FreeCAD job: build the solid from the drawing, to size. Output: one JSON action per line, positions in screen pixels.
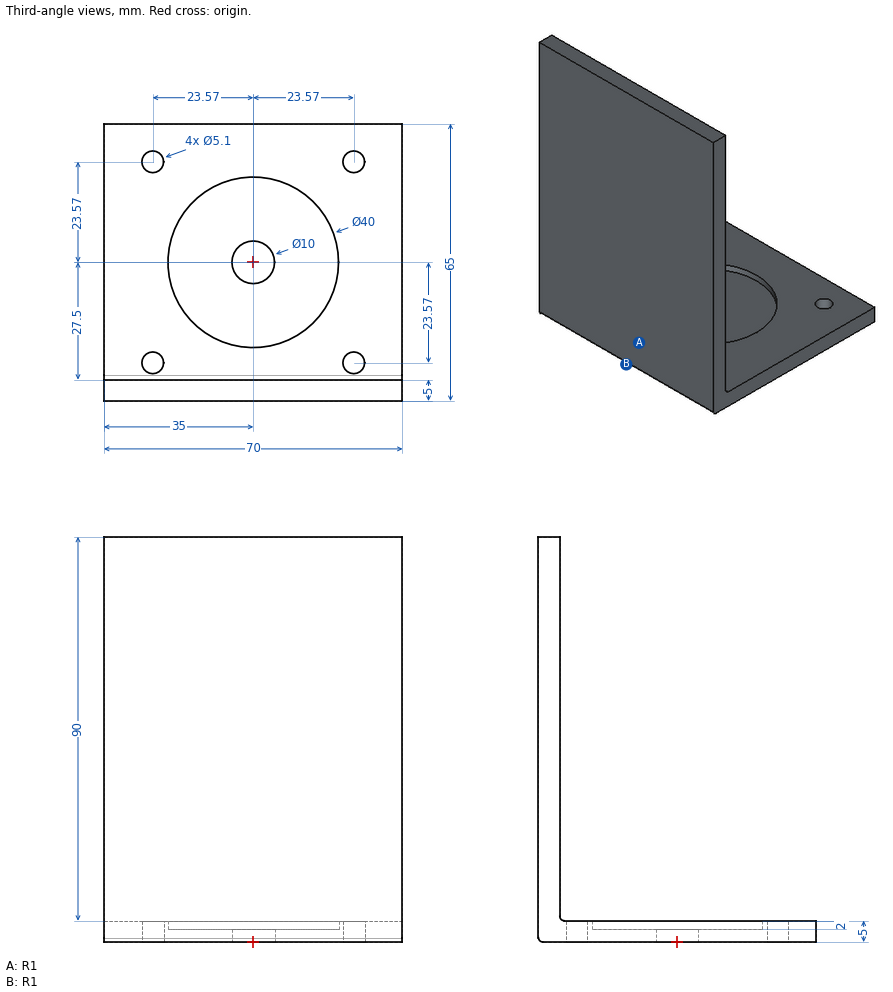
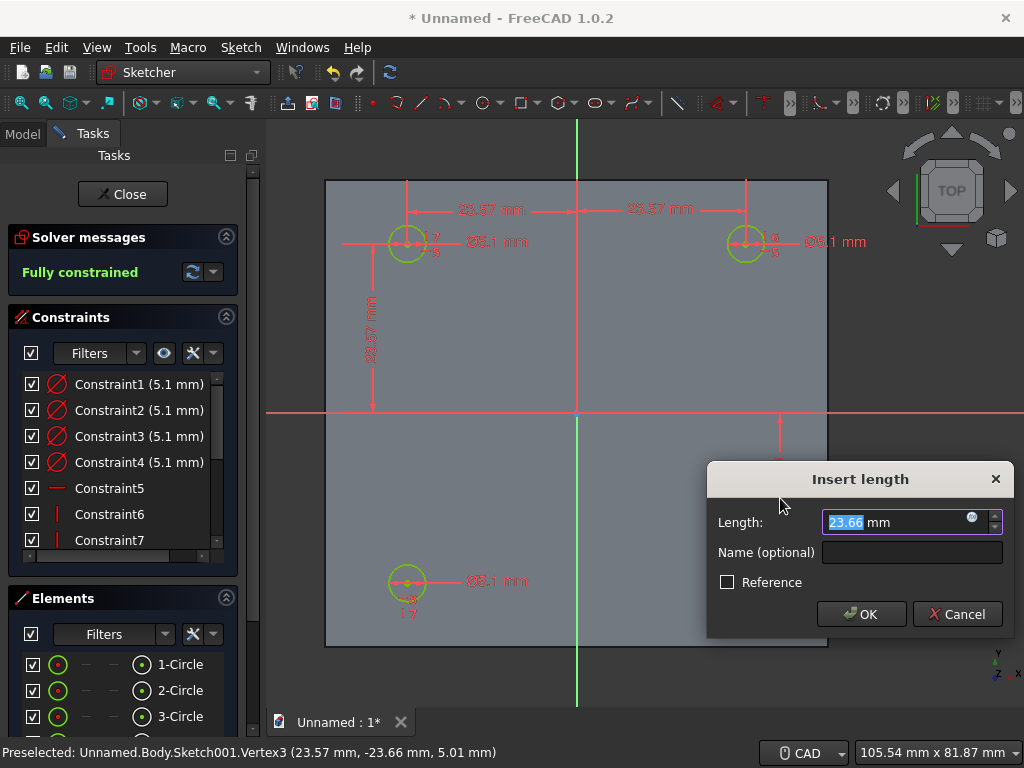
{"action": "type", "text": "23.57"}
{"action": "key", "text": "Return"}
{"action": "key", "text": "Escape"}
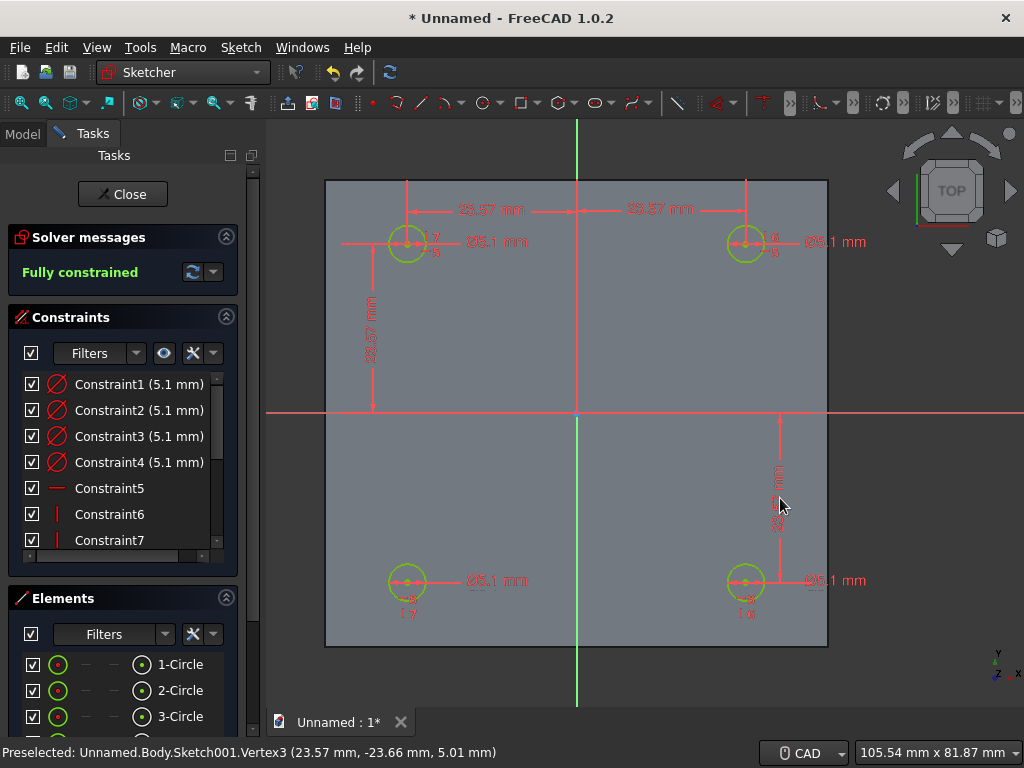
{"action": "left_click", "coordinate": [123, 194]}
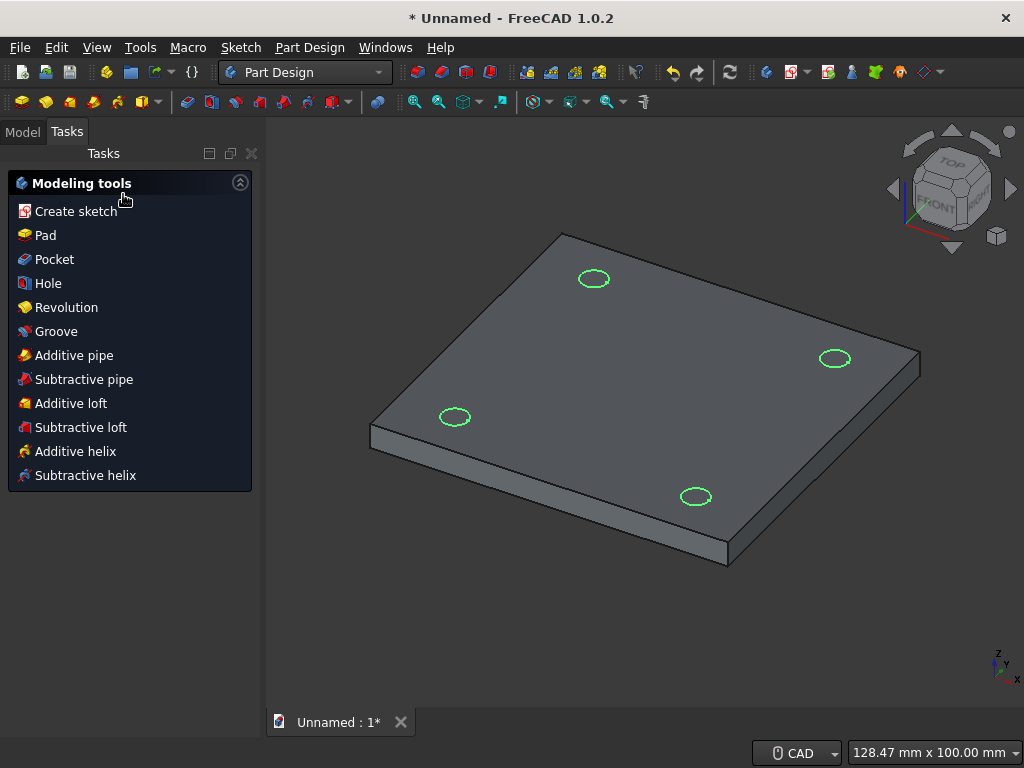
{"action": "left_click", "coordinate": [188, 102]}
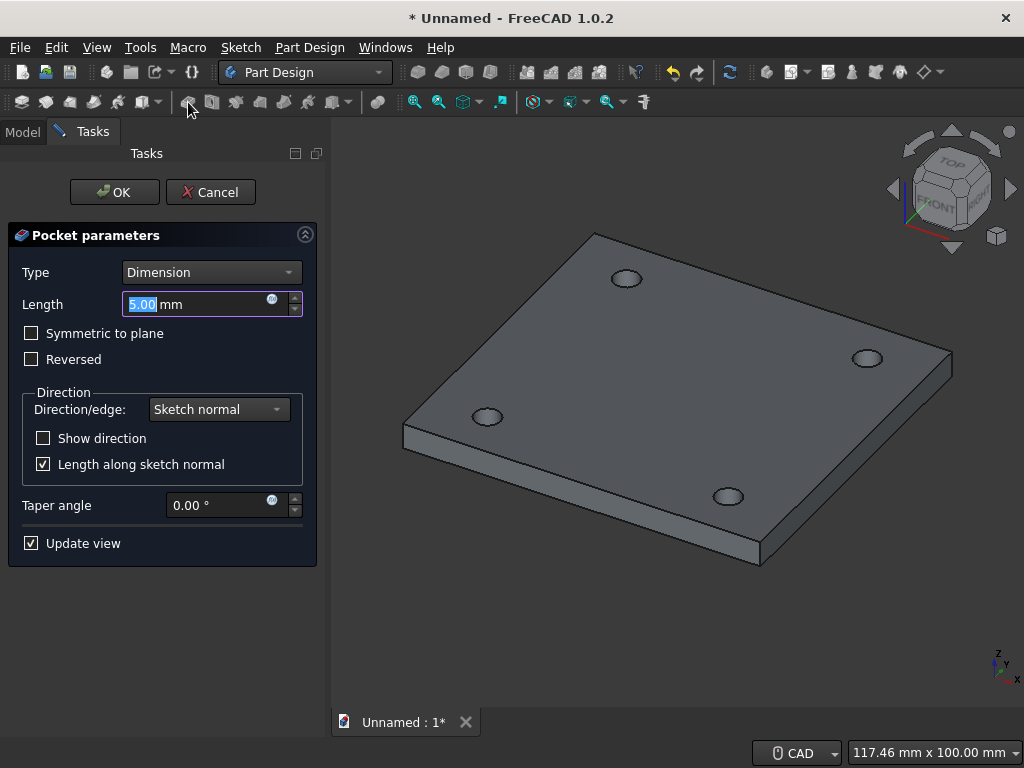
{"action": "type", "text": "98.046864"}
{"action": "key", "text": "Tab"}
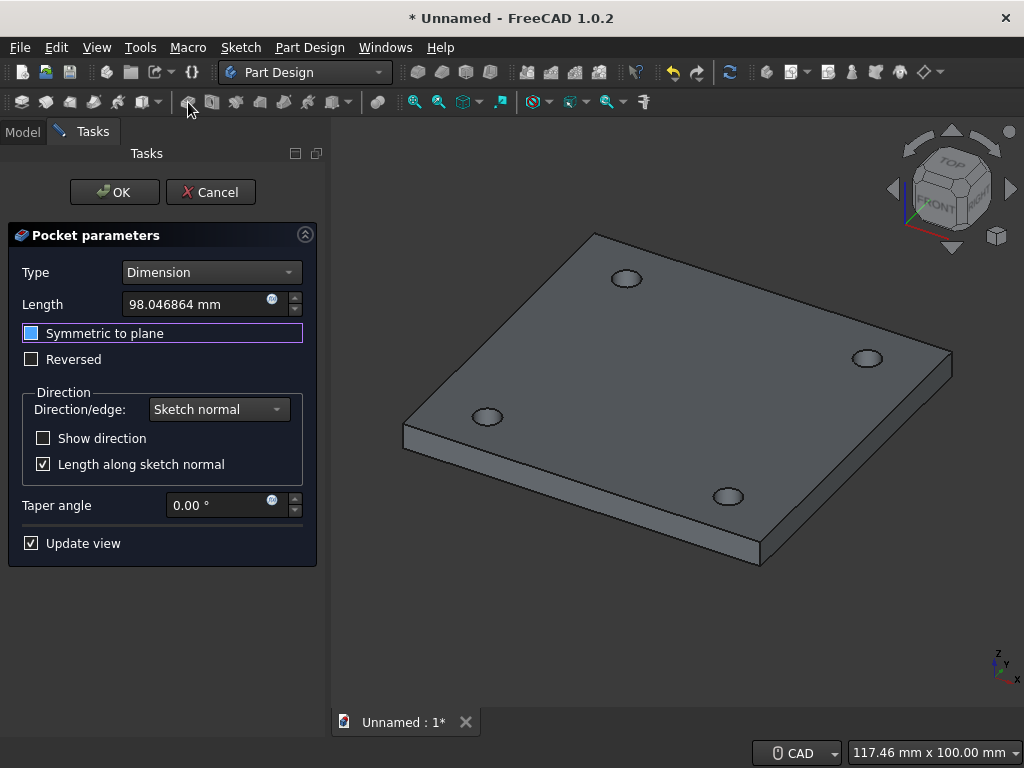
{"action": "left_click", "coordinate": [30, 333]}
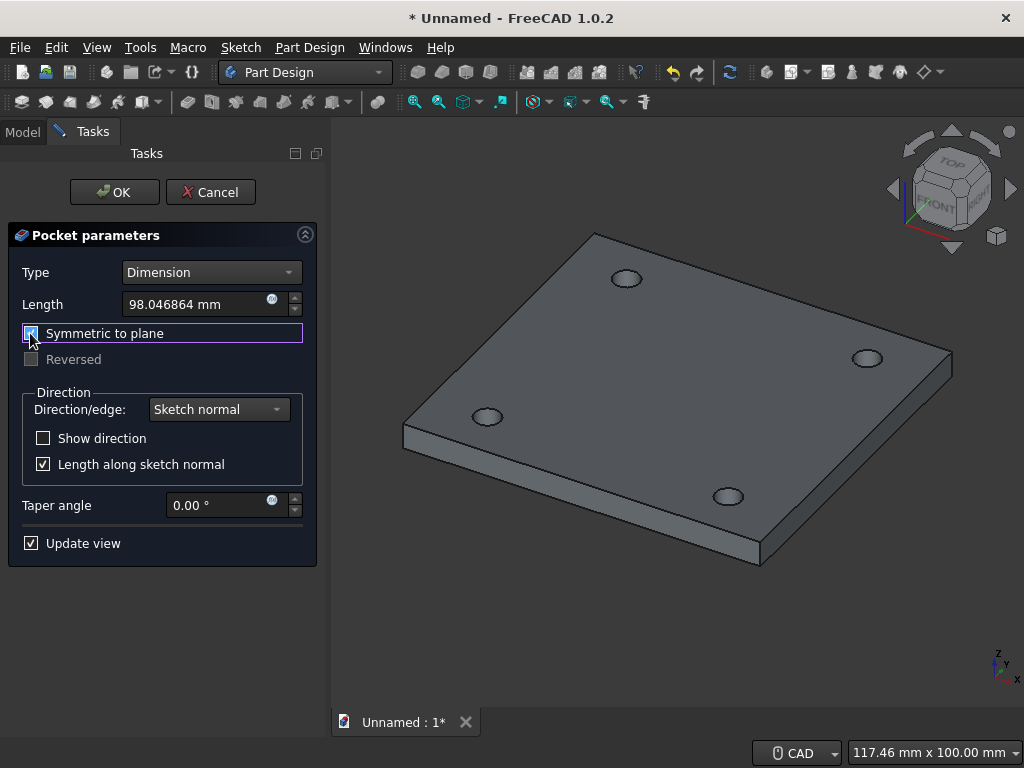
{"action": "left_click", "coordinate": [115, 192]}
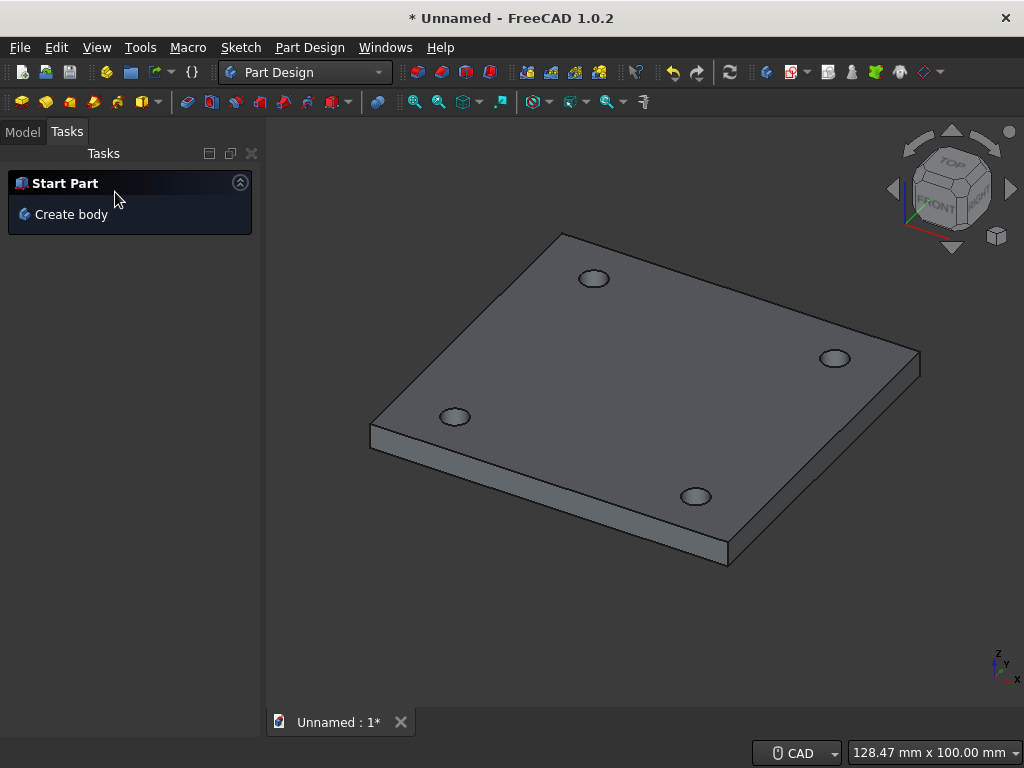
{"action": "left_click", "coordinate": [645, 387]}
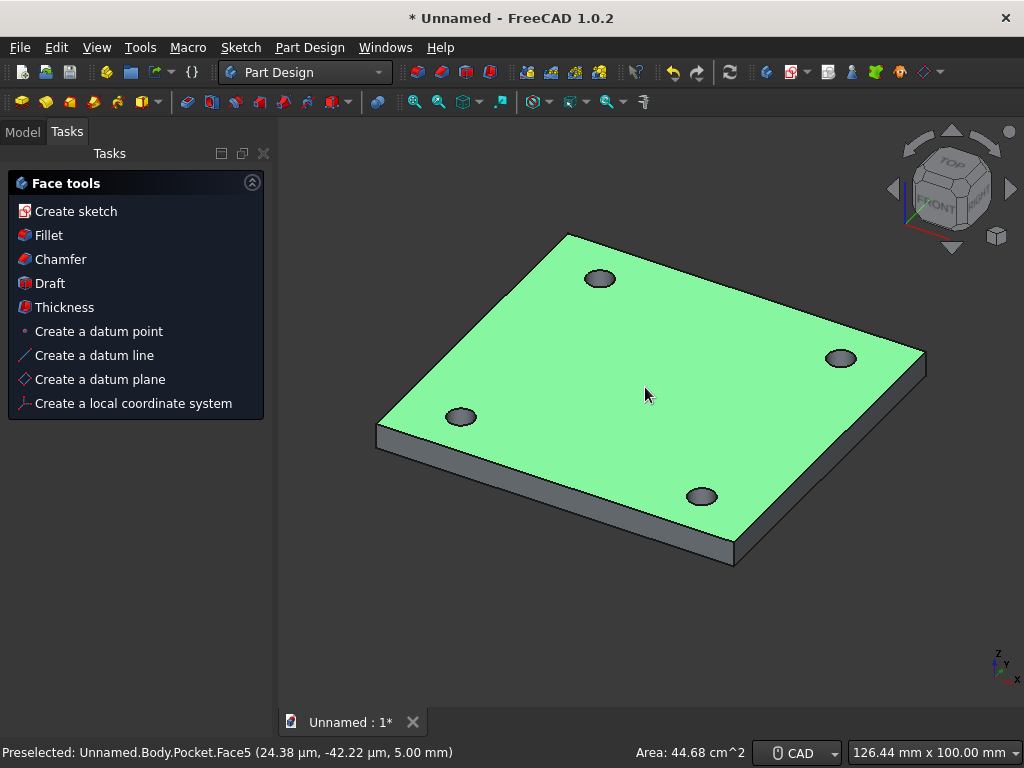
{"action": "left_click", "coordinate": [792, 72]}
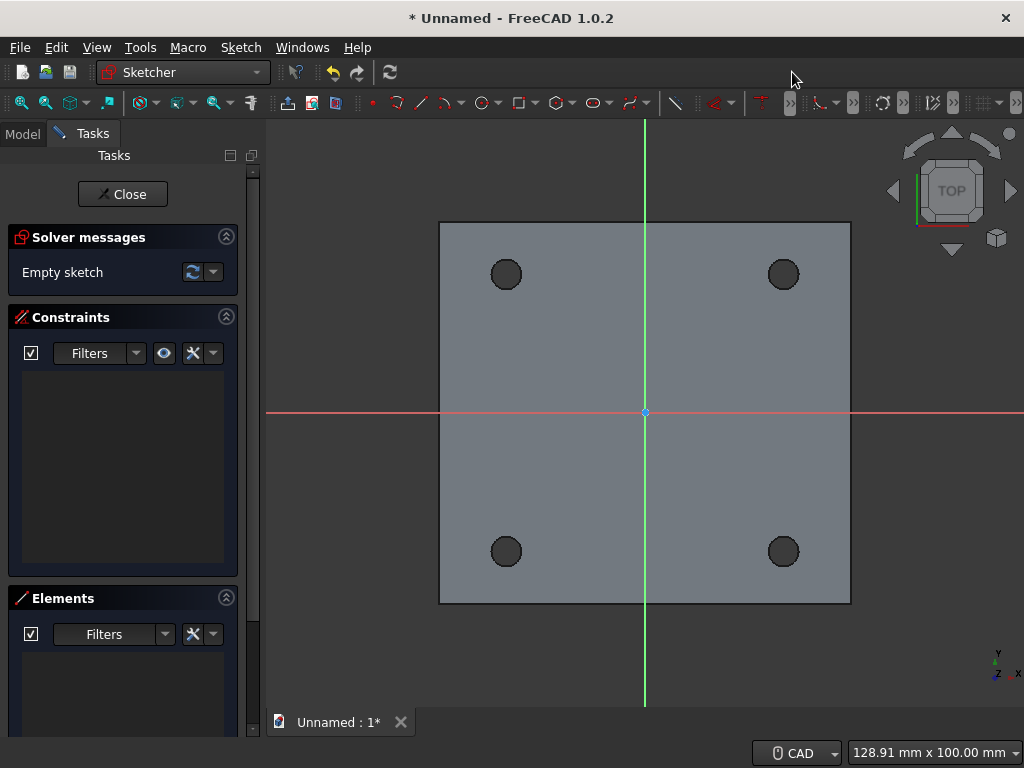
{"action": "scroll", "coordinate": [294, 147], "scroll_direction": "down", "scroll_amount": 1}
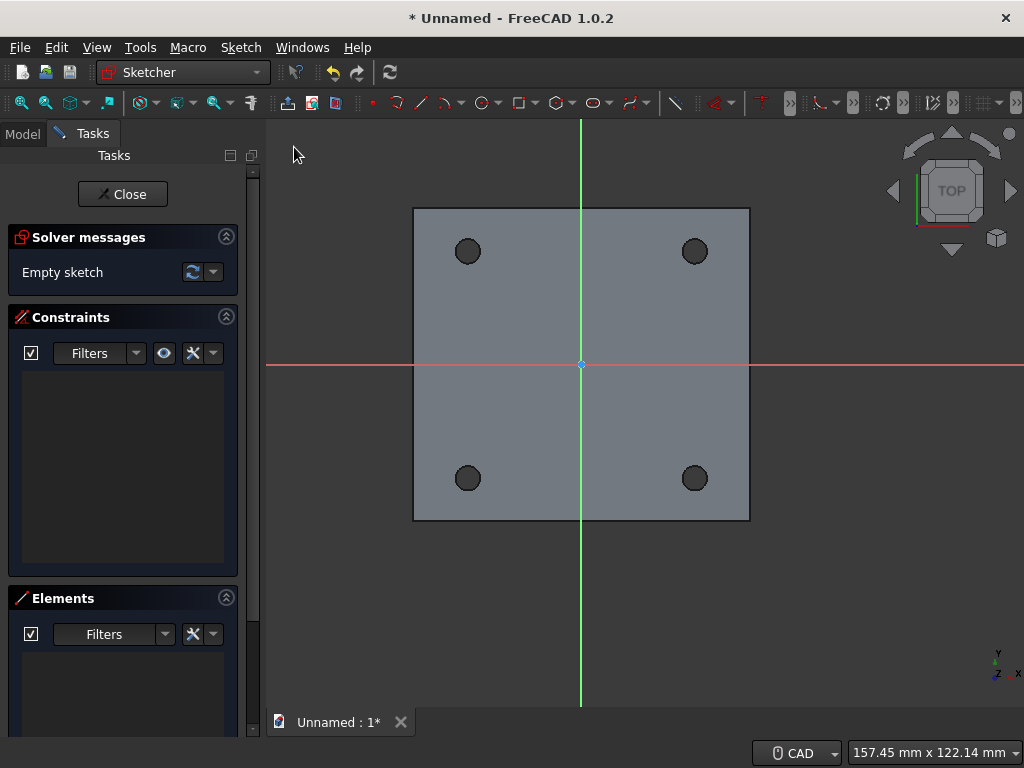
{"action": "left_click", "coordinate": [520, 104]}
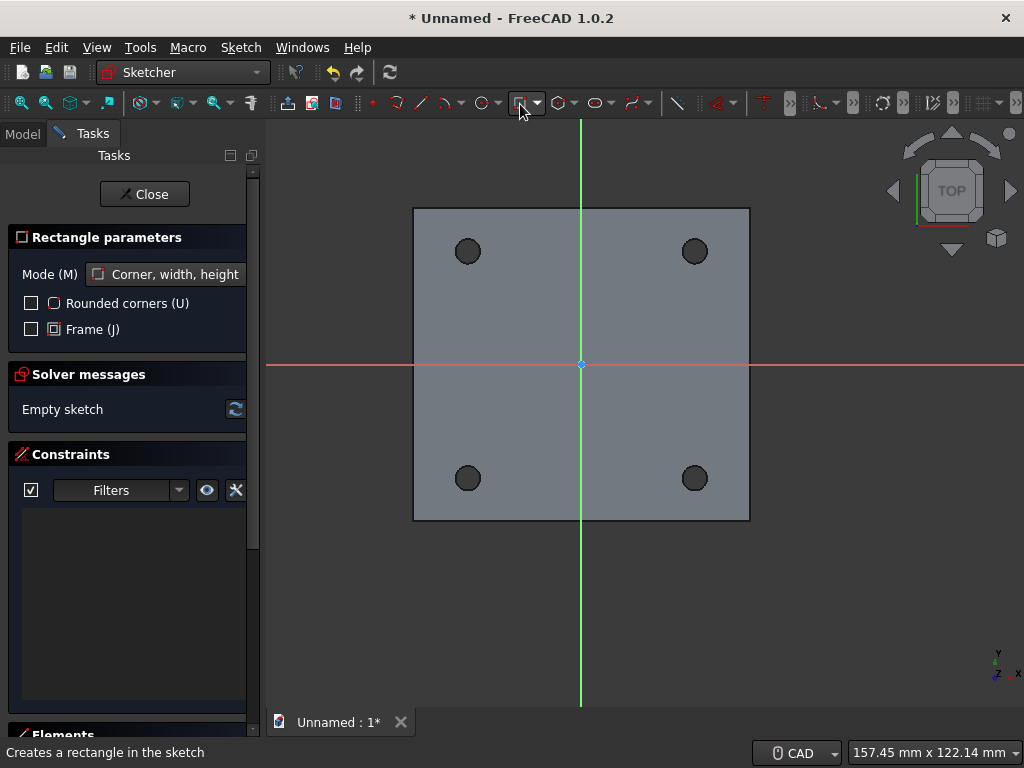
{"action": "left_click", "coordinate": [413, 497]}
{"action": "mouse_move", "coordinate": [750, 521]}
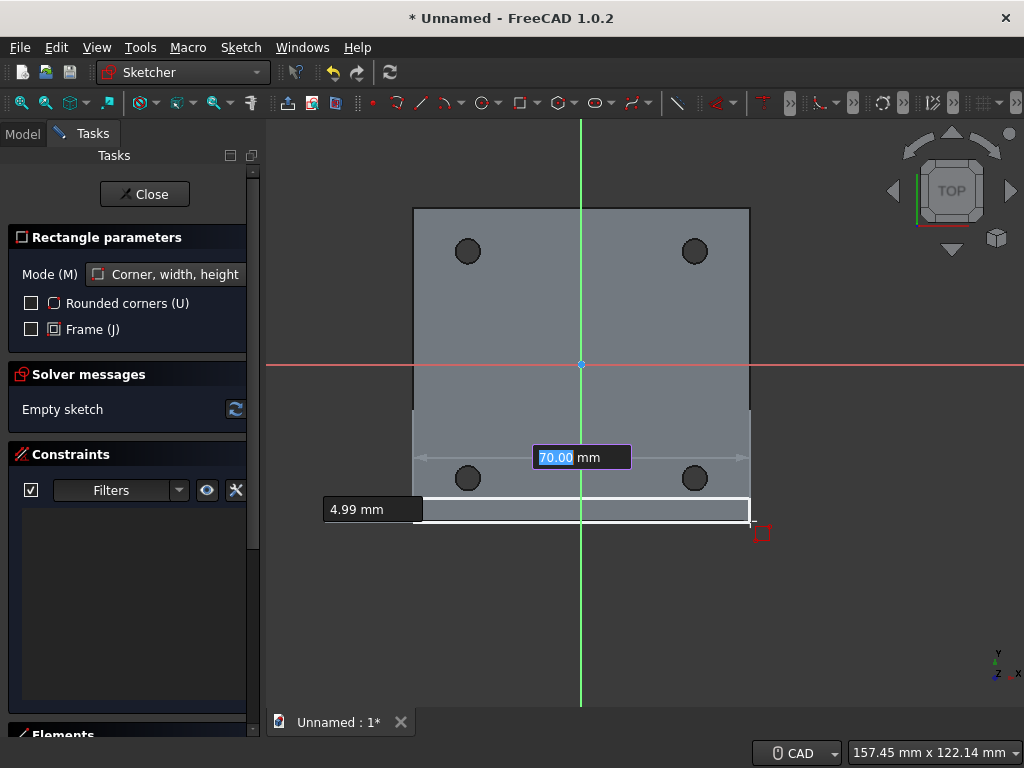
{"action": "type", "text": "70"}
{"action": "key", "text": "Tab"}
{"action": "type", "text": "5"}
{"action": "key", "text": "Return"}
{"action": "key", "text": "Escape"}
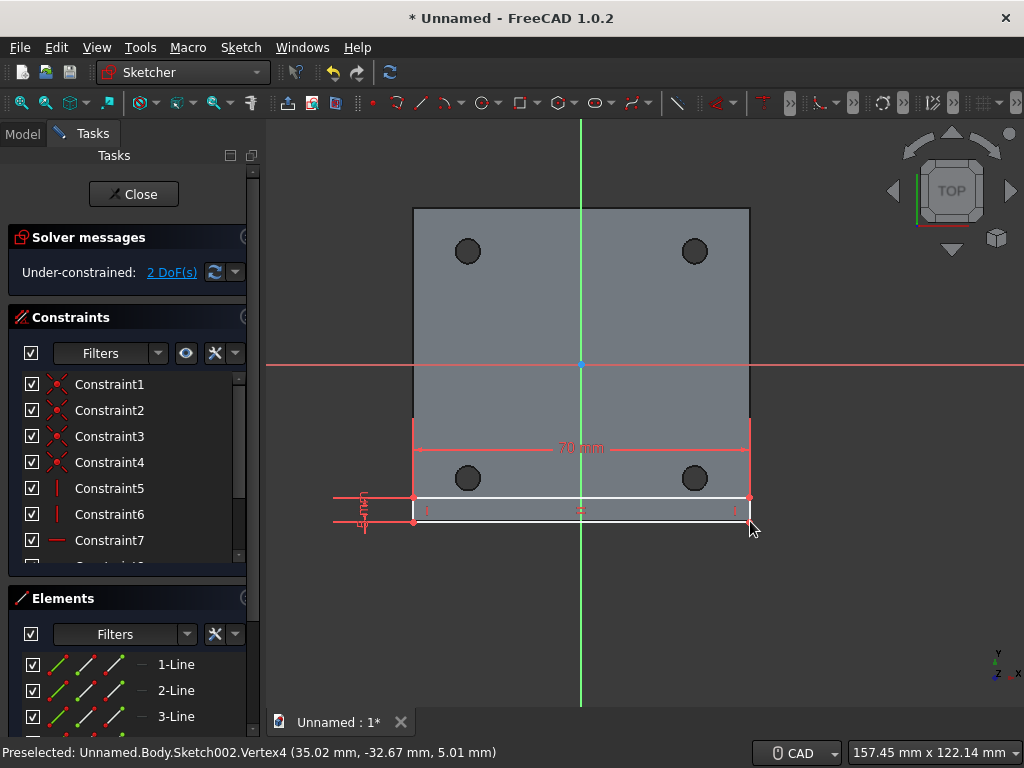
{"action": "left_click", "coordinate": [716, 104]}